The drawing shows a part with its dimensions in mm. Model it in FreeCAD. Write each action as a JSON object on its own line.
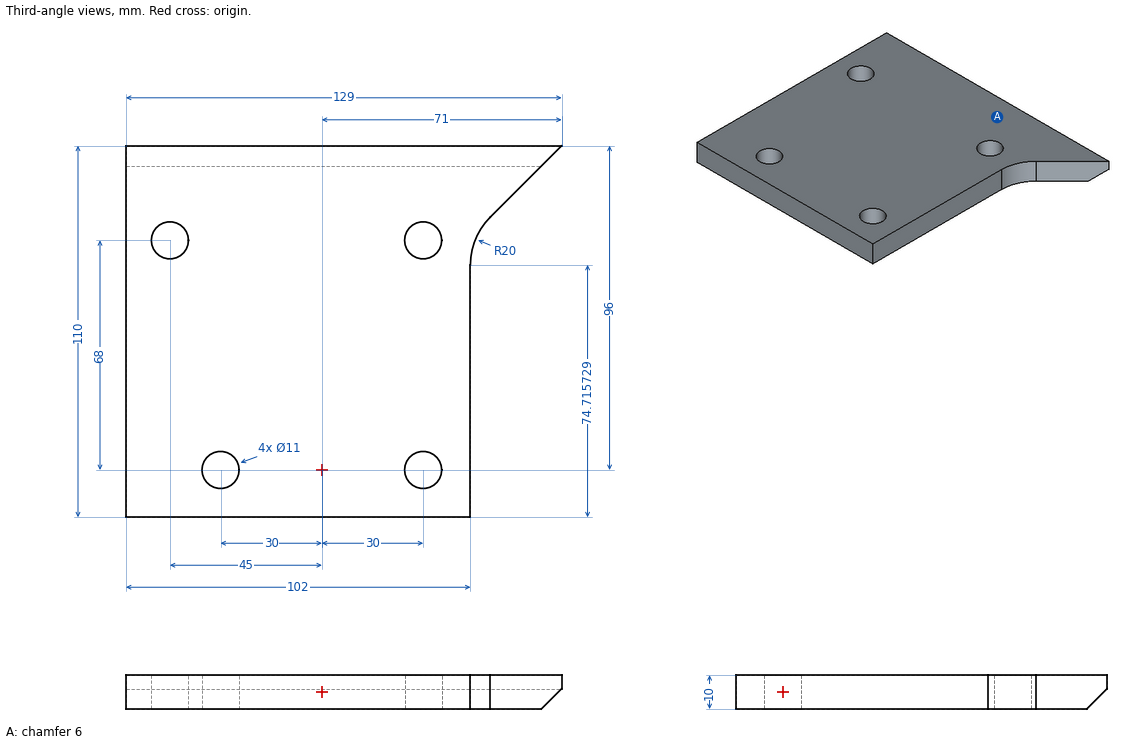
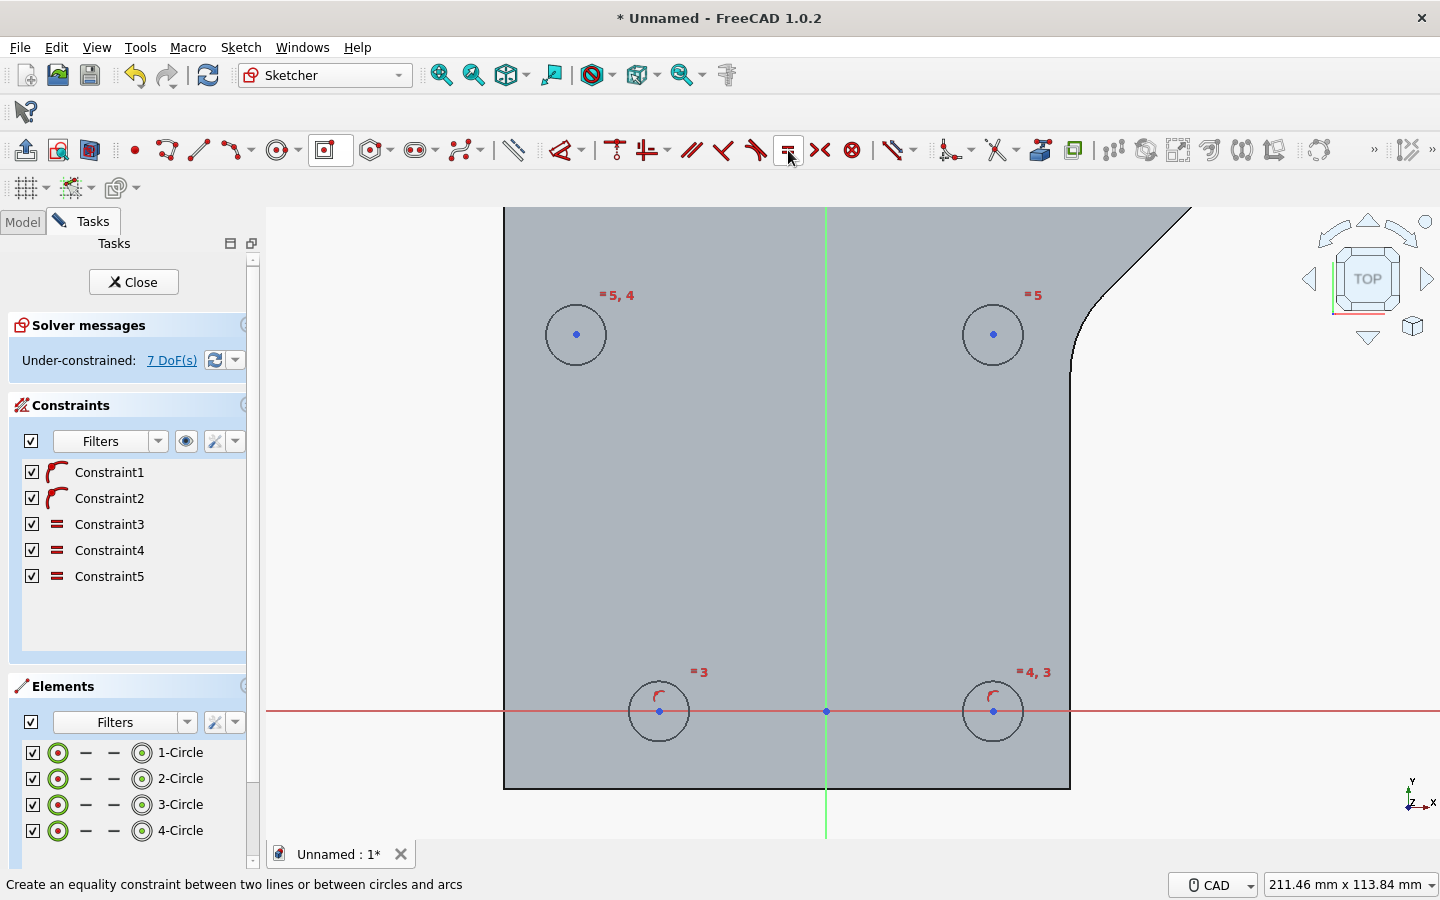
{"action": "left_click", "coordinate": [560, 150]}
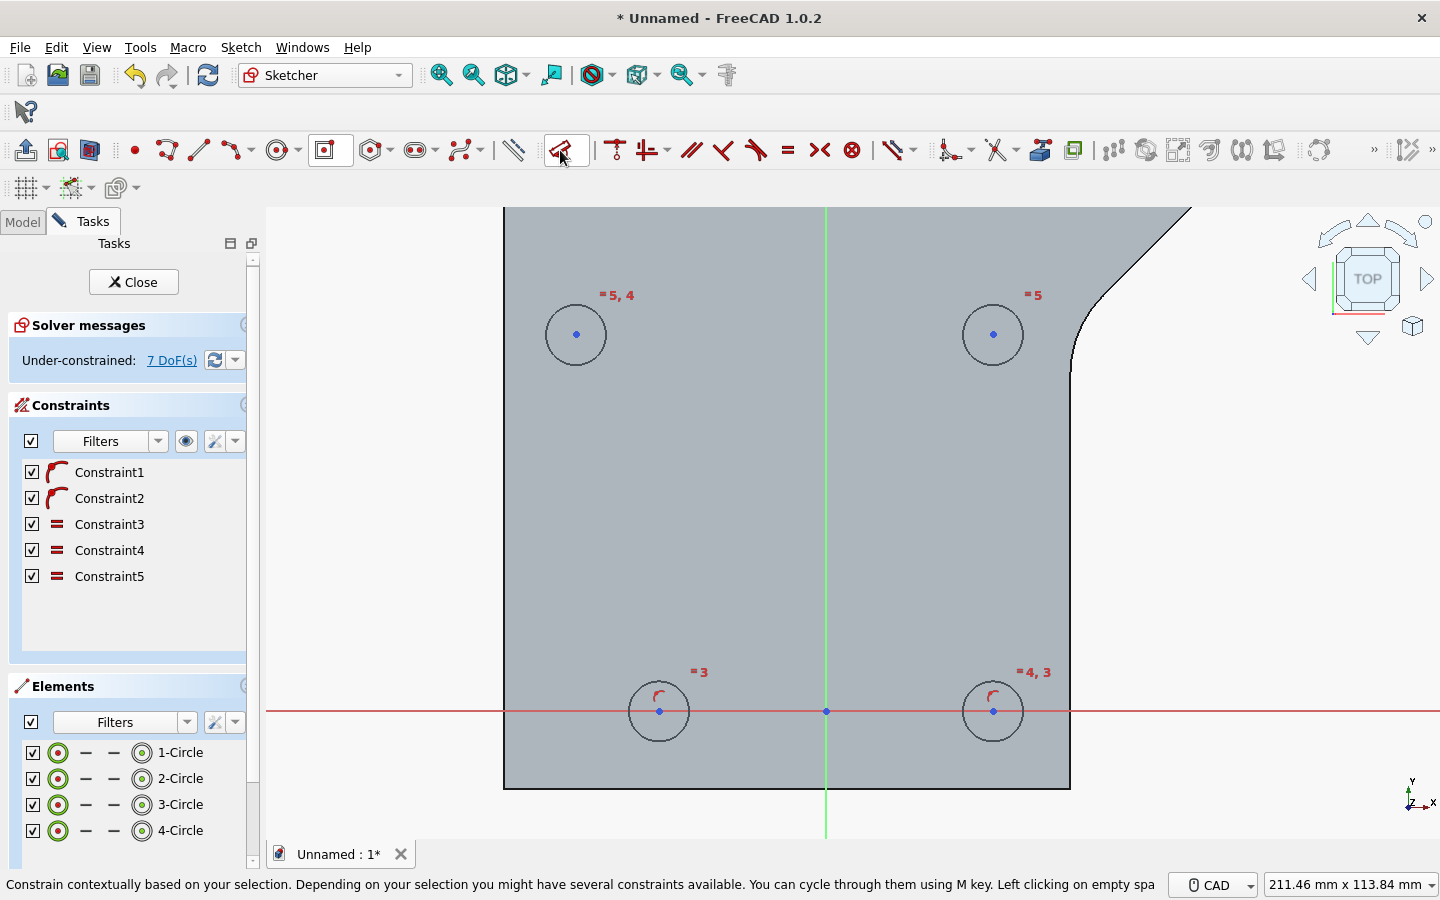
{"action": "left_click", "coordinate": [680, 690]}
{"action": "left_click", "coordinate": [702, 667]}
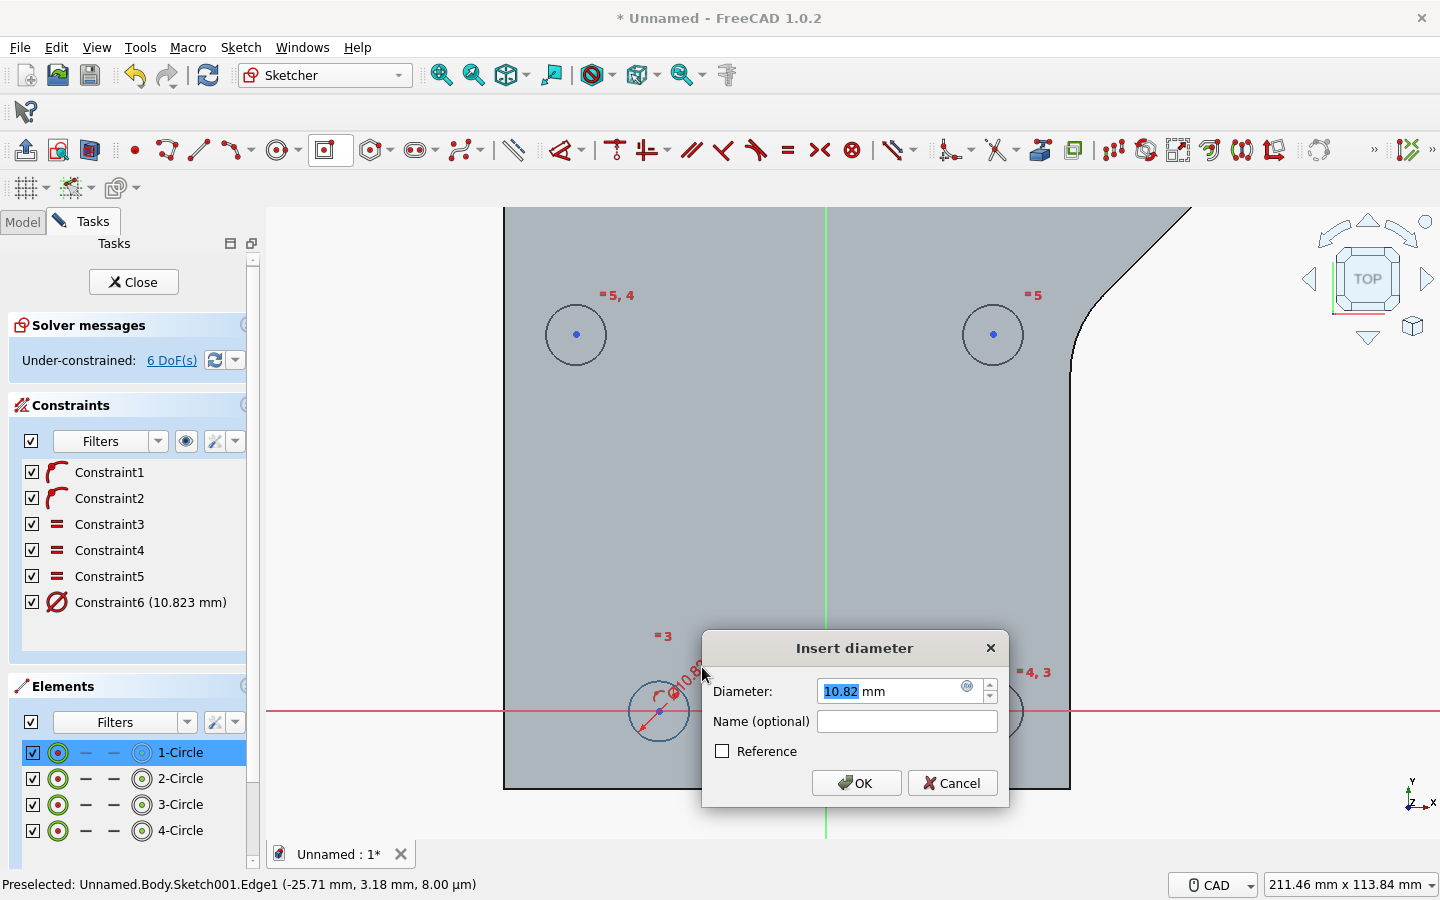
{"action": "type", "text": "11"}
{"action": "key", "text": "Return"}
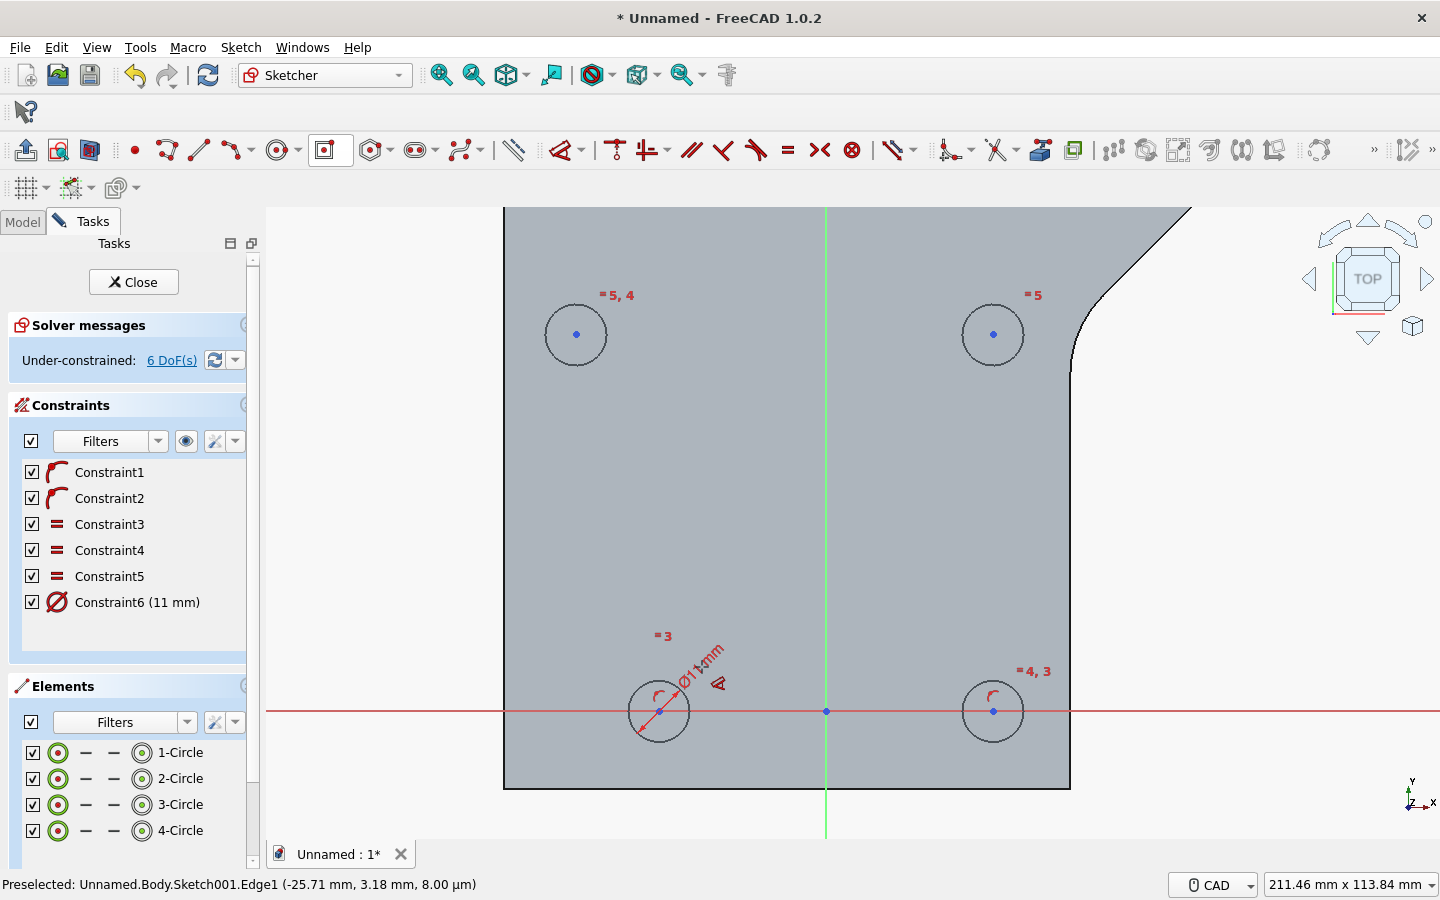
{"action": "left_click", "coordinate": [659, 711]}
{"action": "left_click", "coordinate": [743, 745]}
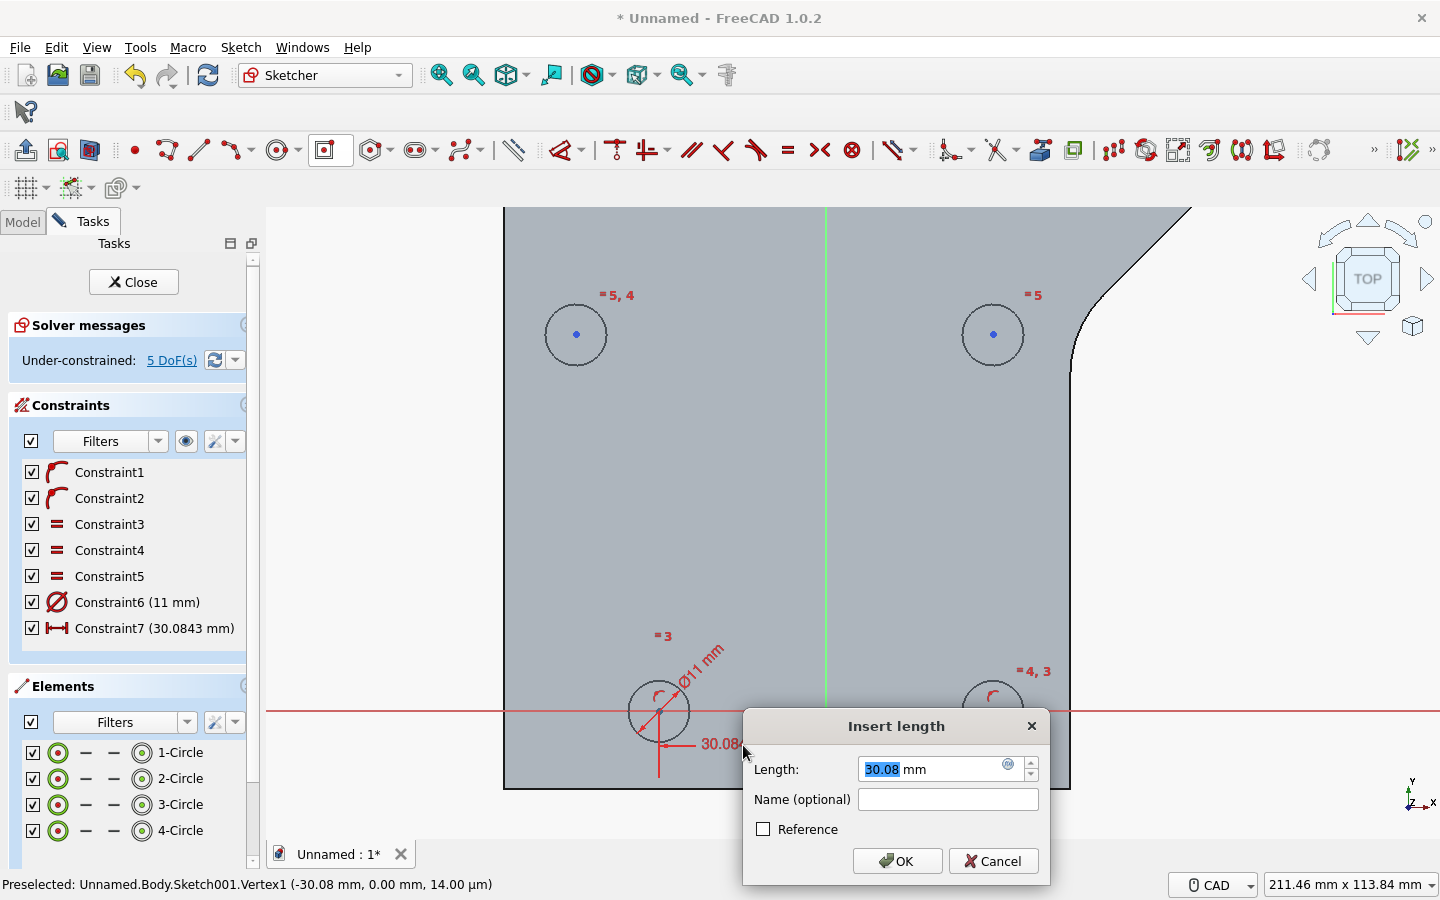
{"action": "type", "text": "30"}
{"action": "key", "text": "Return"}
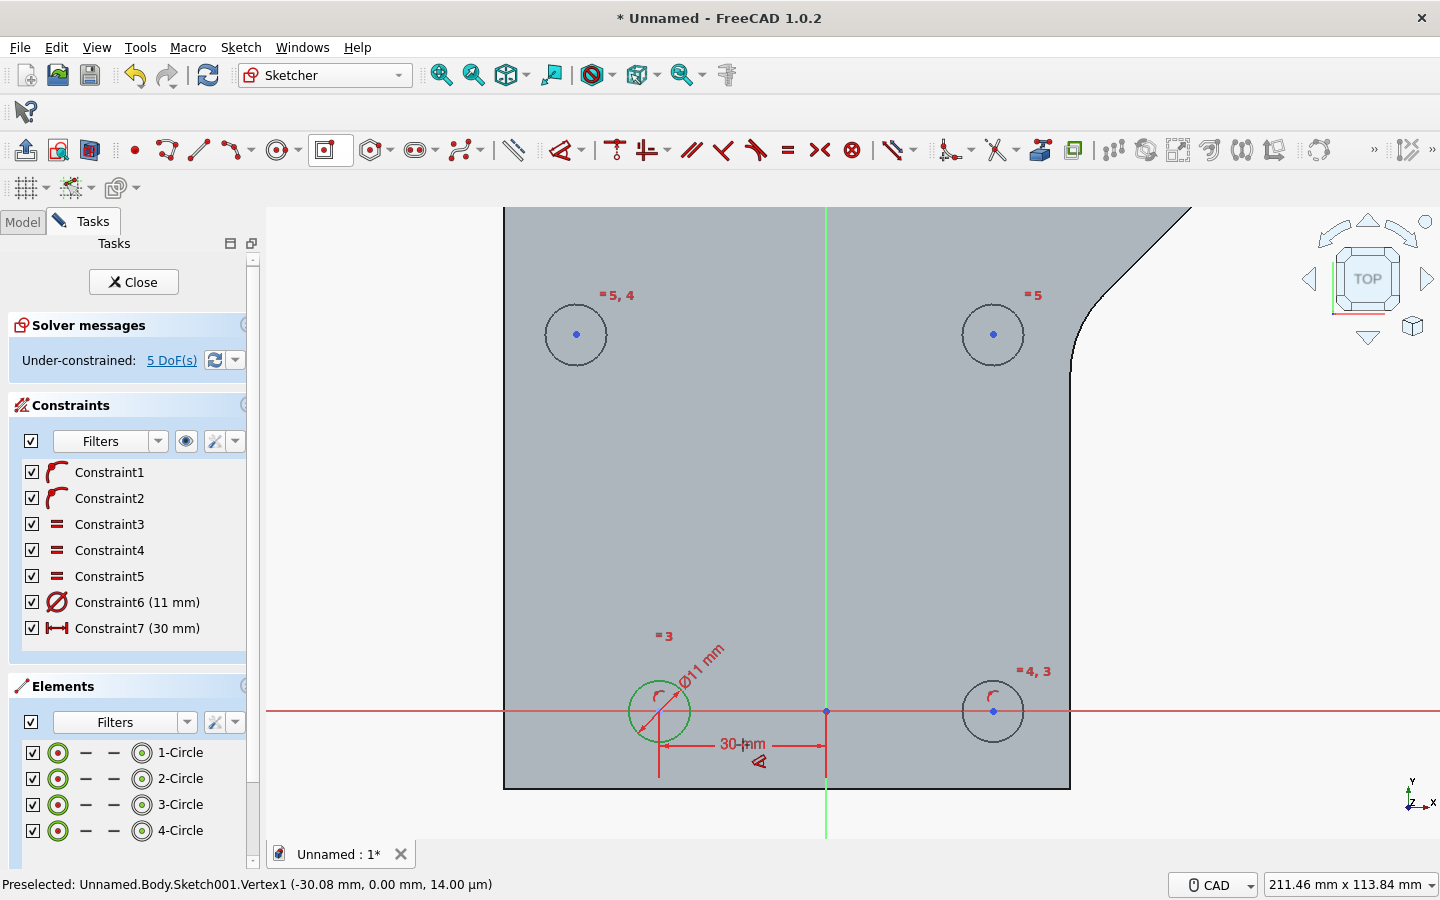
{"action": "left_click", "coordinate": [993, 711]}
{"action": "left_click", "coordinate": [910, 745]}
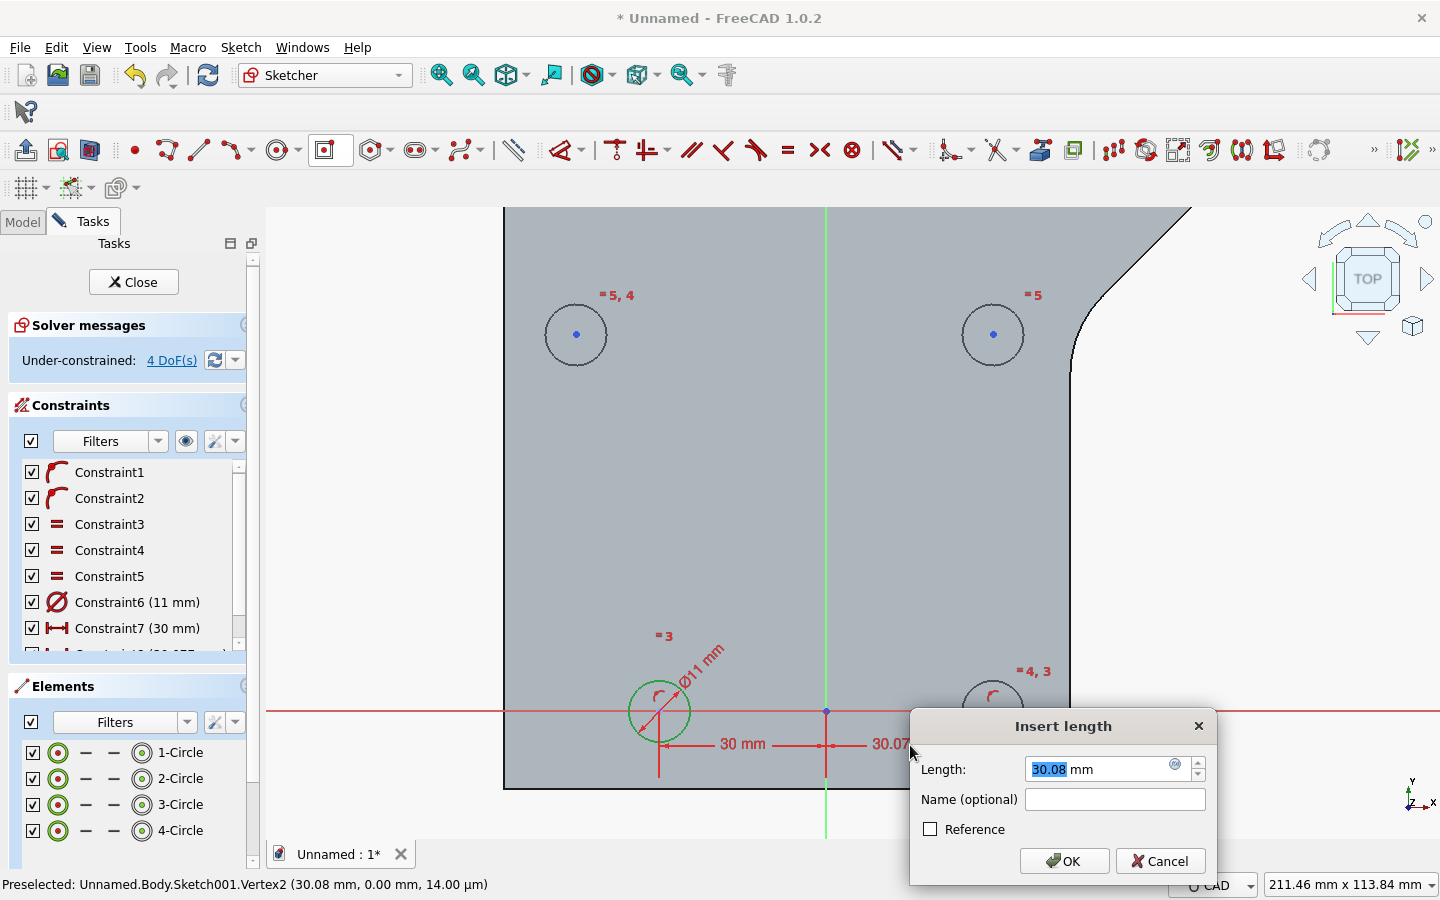
{"action": "type", "text": "30"}
{"action": "key", "text": "Return"}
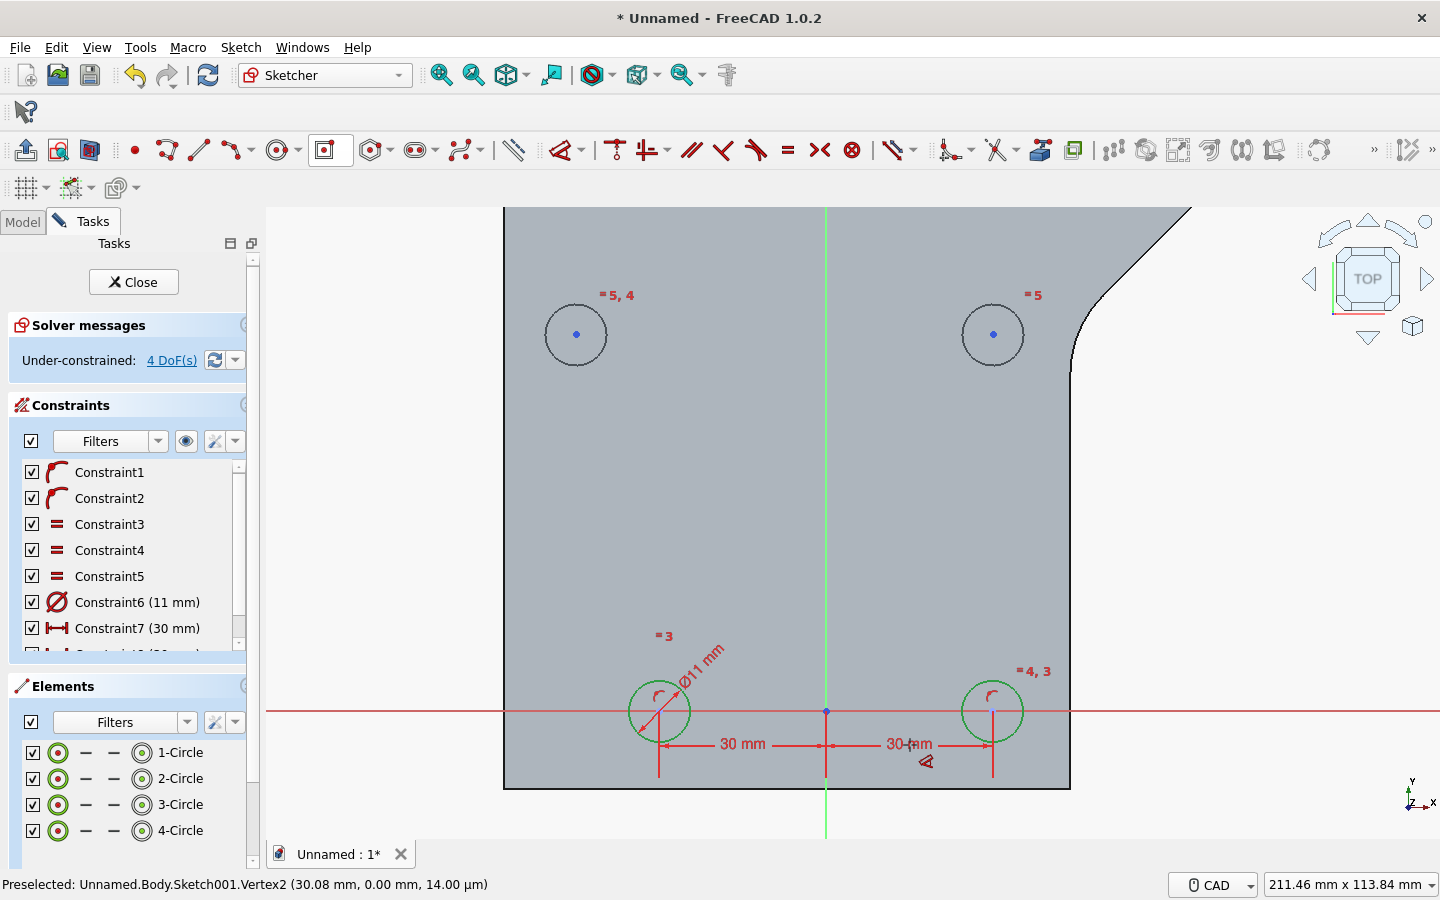
{"action": "left_click", "coordinate": [576, 335]}
{"action": "left_click", "coordinate": [614, 745]}